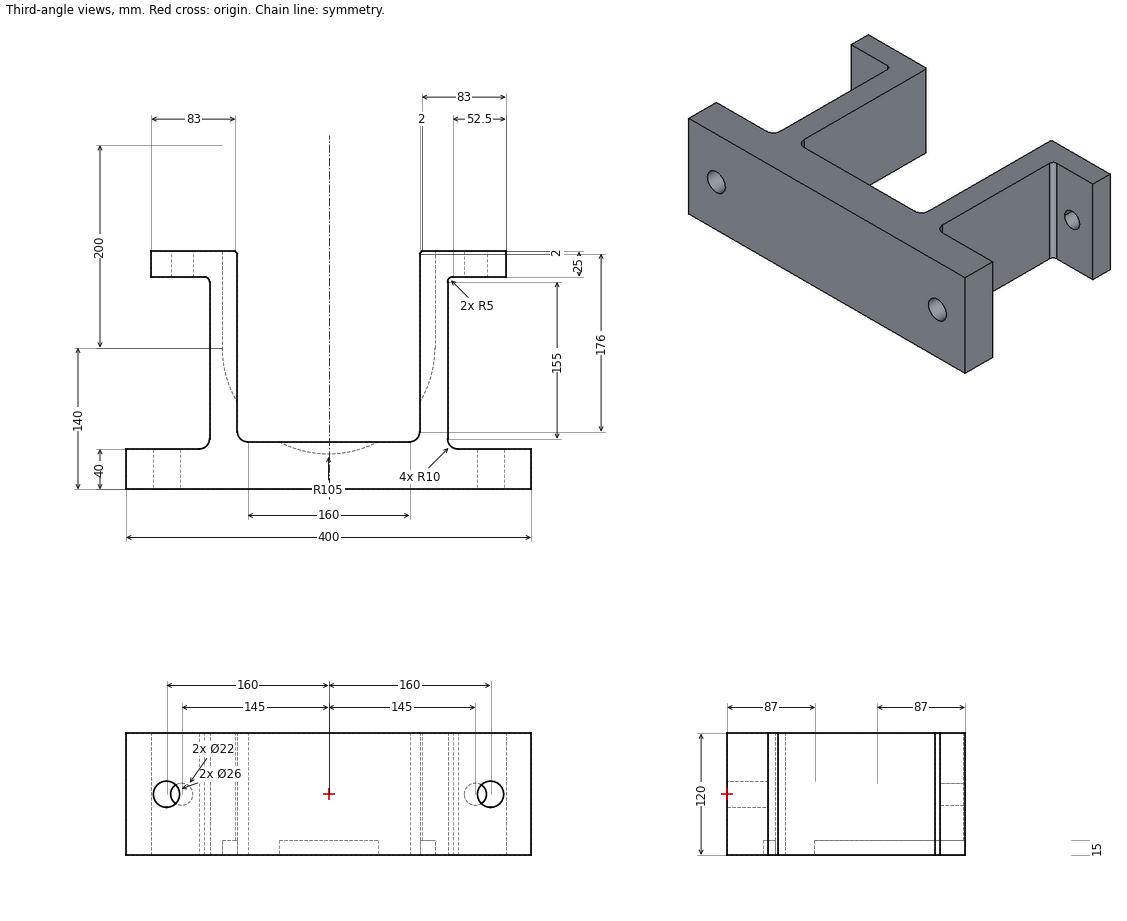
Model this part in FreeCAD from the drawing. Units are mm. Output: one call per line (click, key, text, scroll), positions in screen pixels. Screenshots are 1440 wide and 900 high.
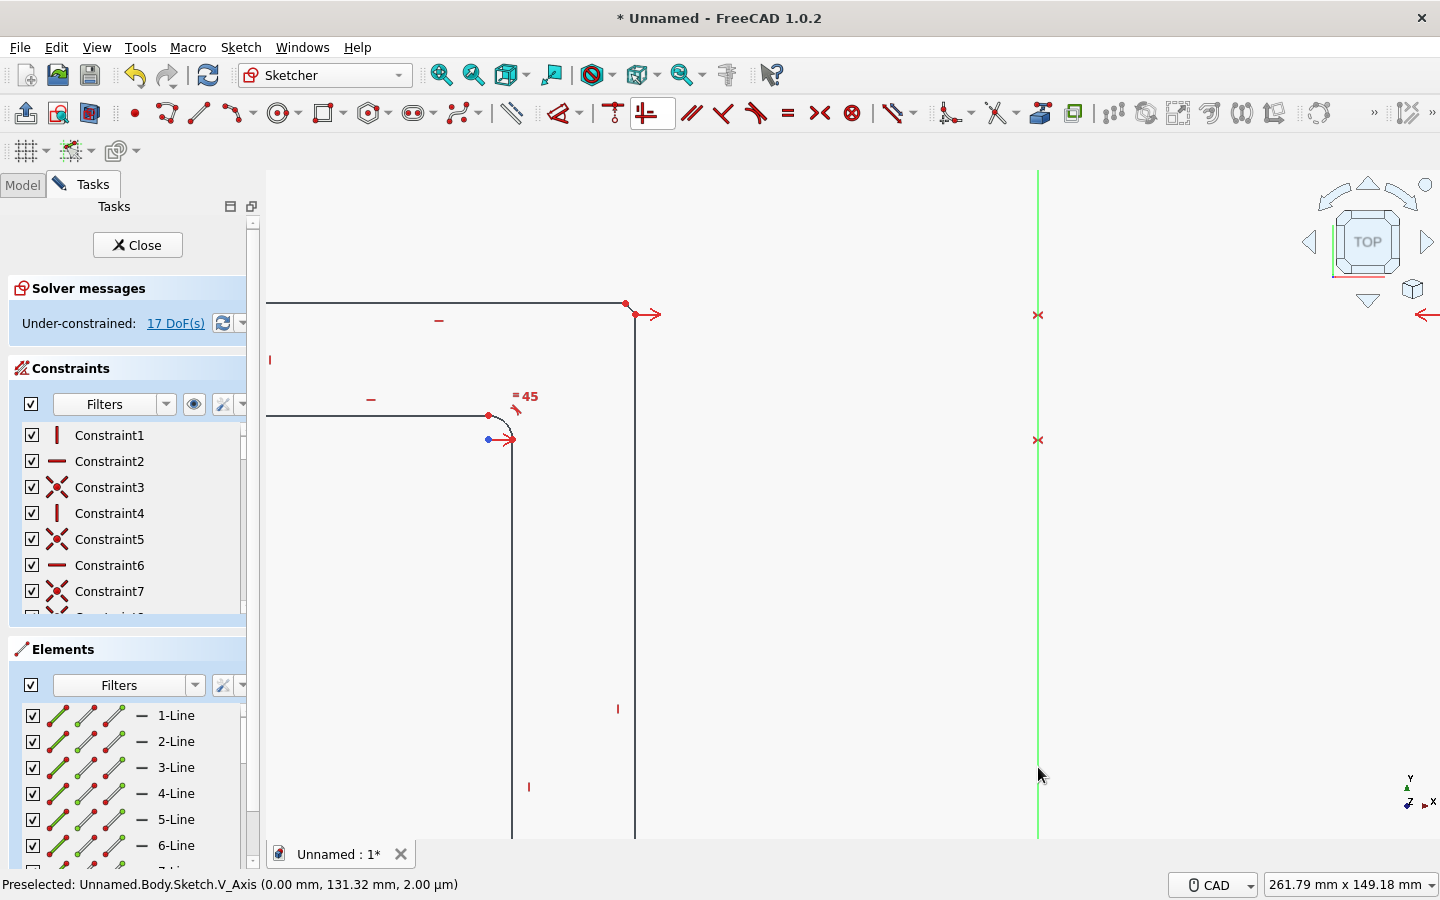
scroll(637, 315, down, 5)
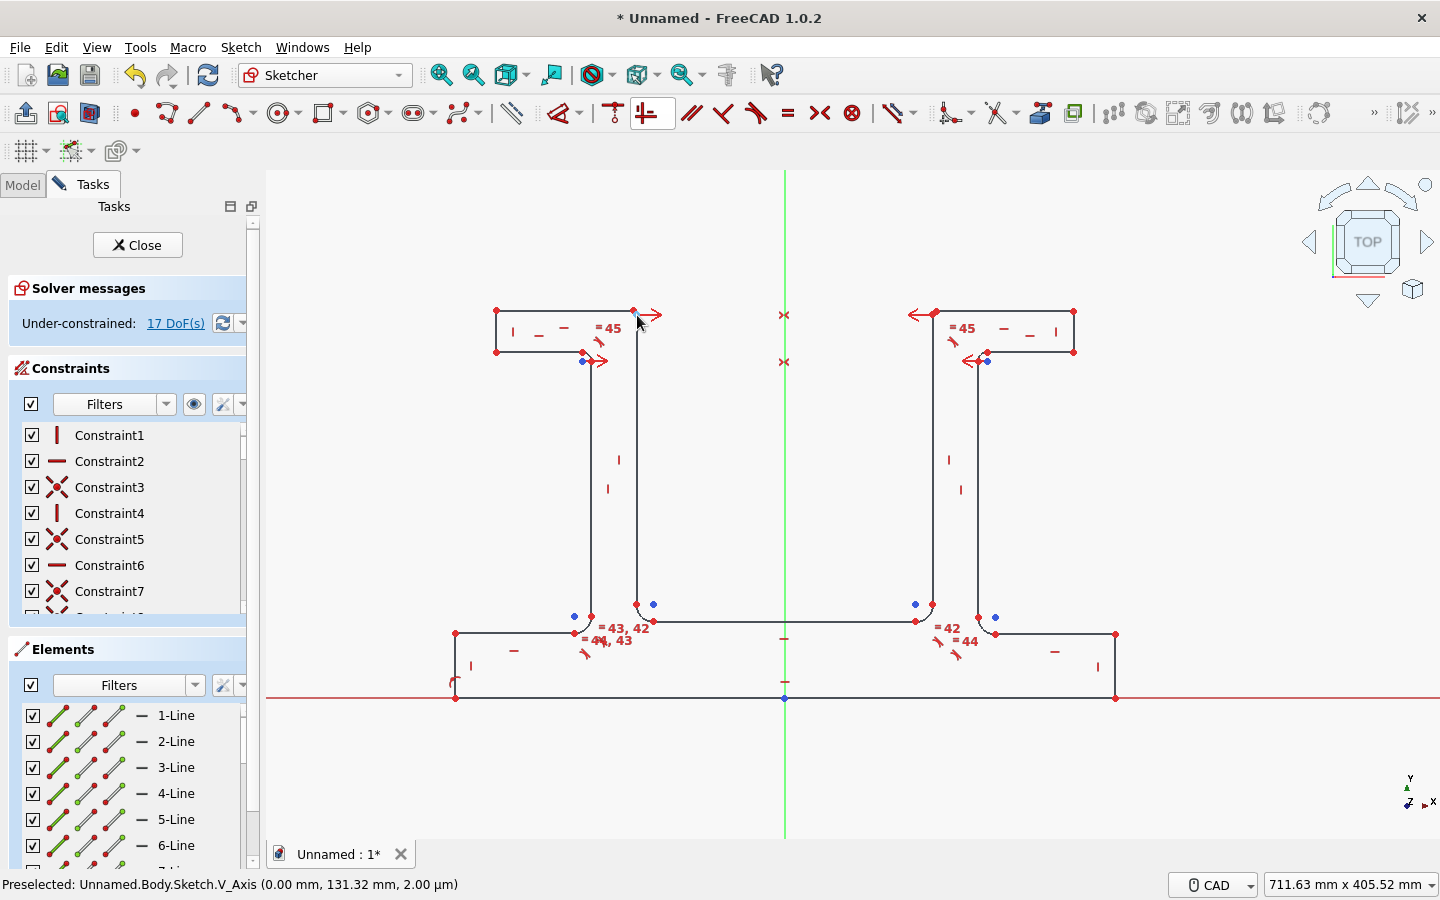
scroll(936, 311, up, 5)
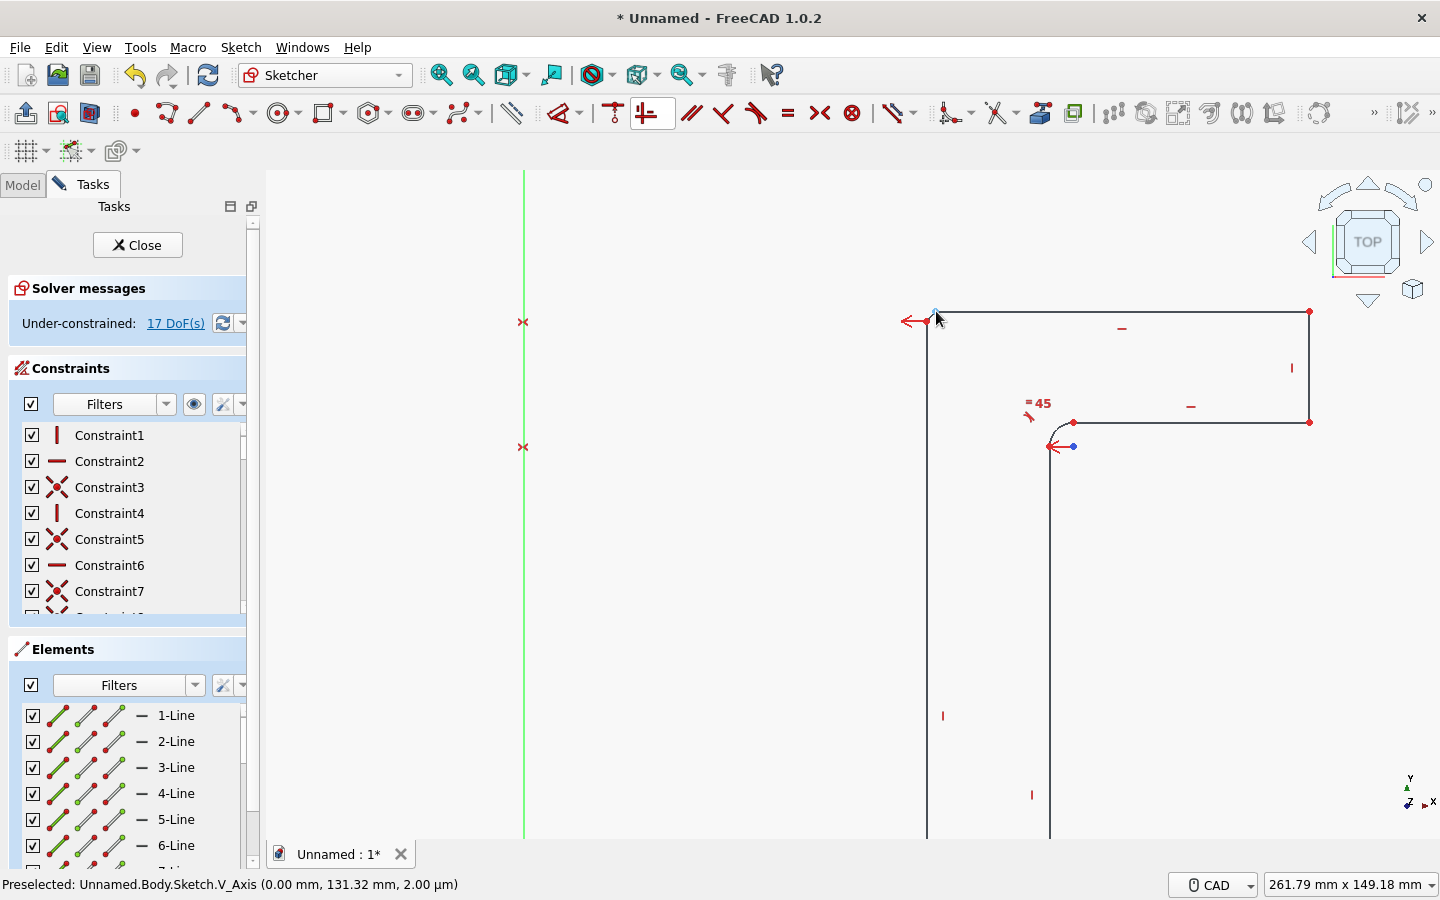
click(936, 312)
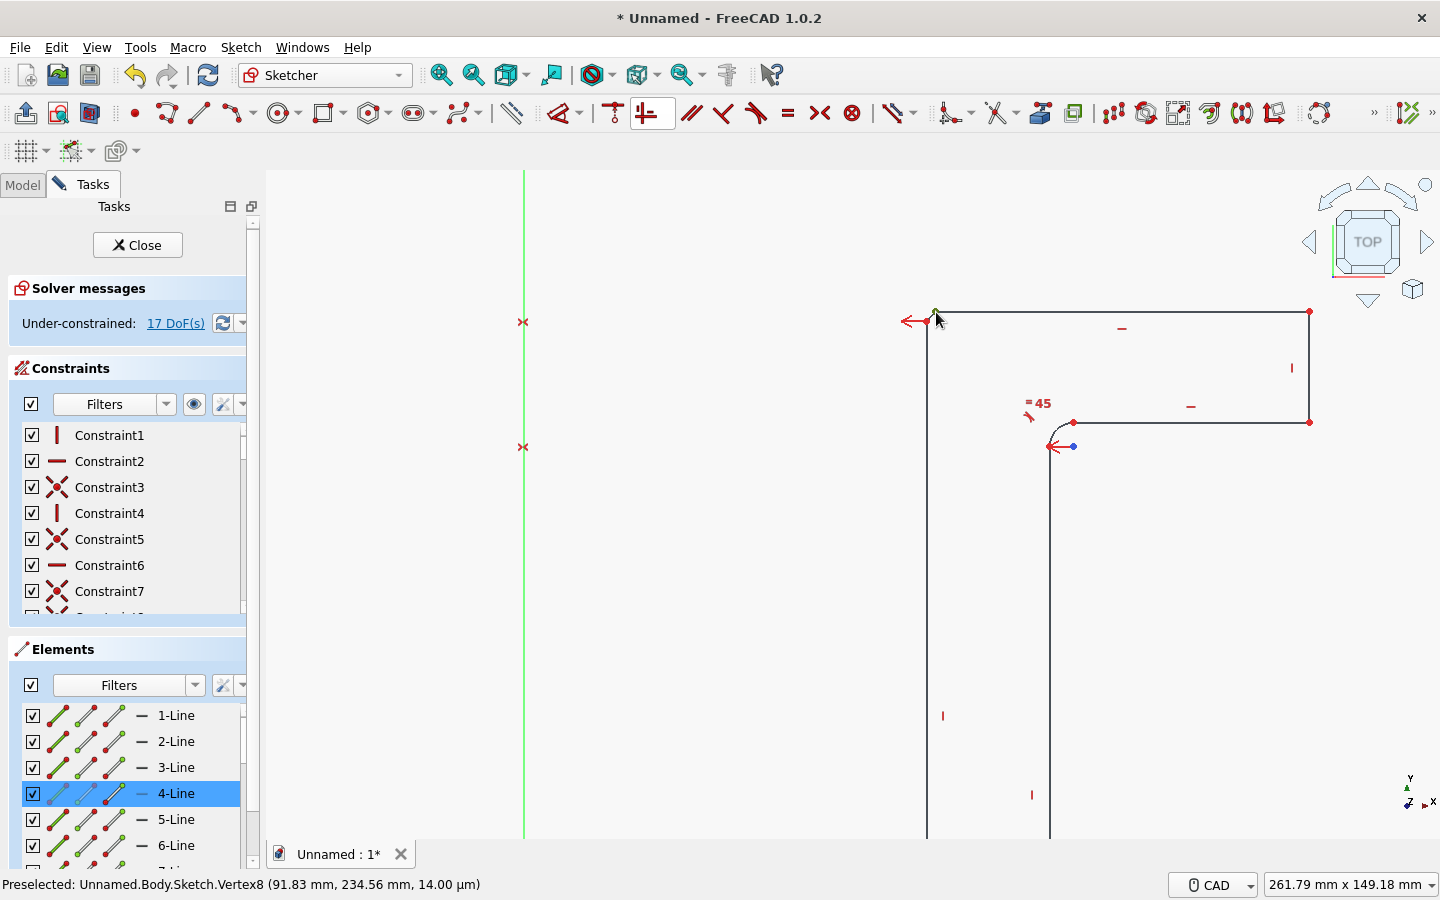
scroll(936, 311, down, 5)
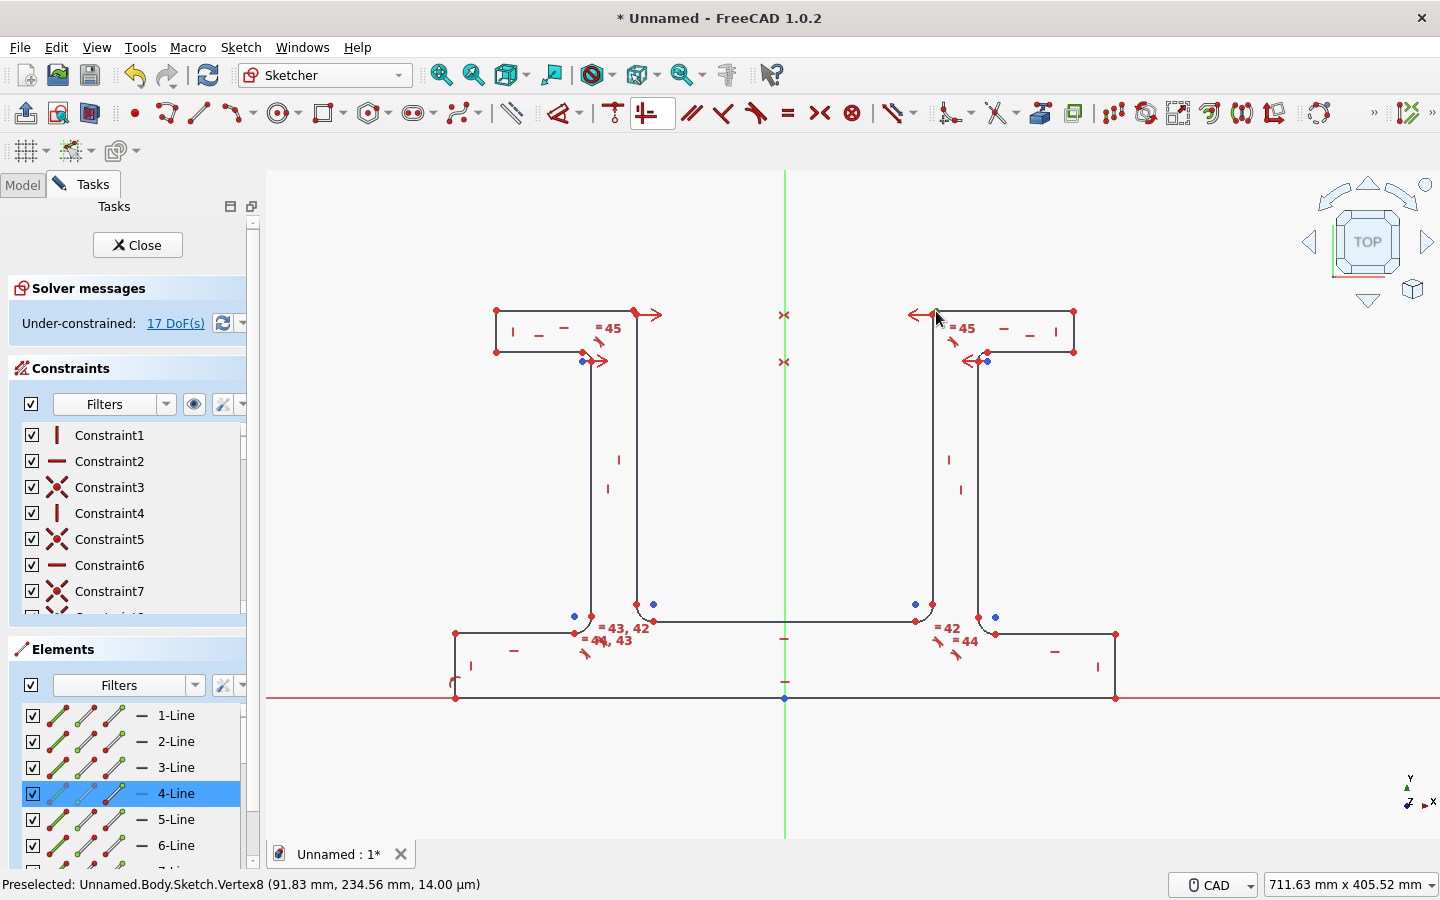
scroll(633, 311, up, 5)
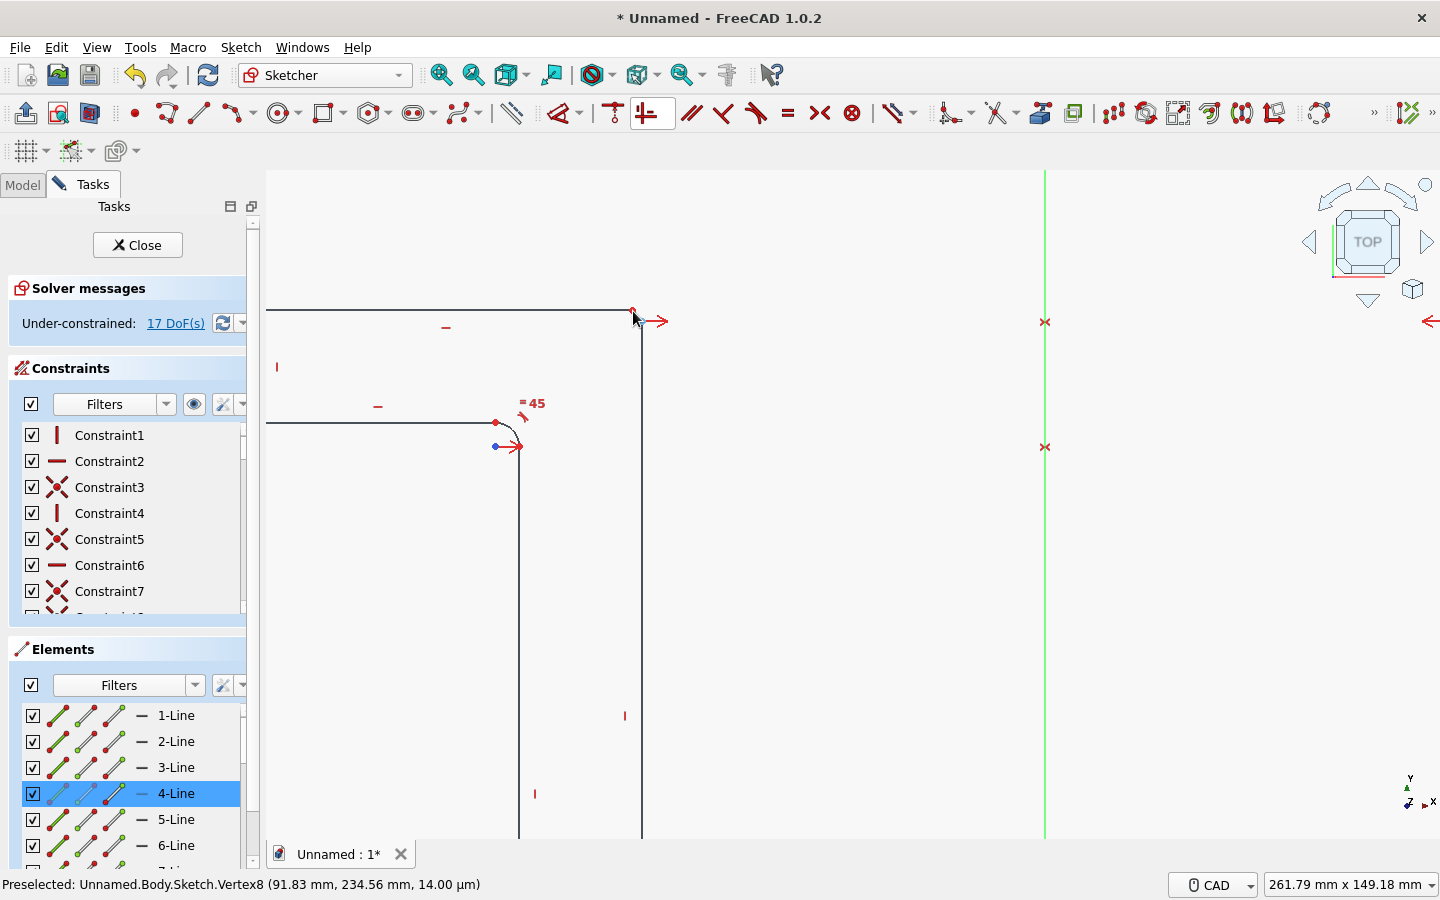
click(633, 310)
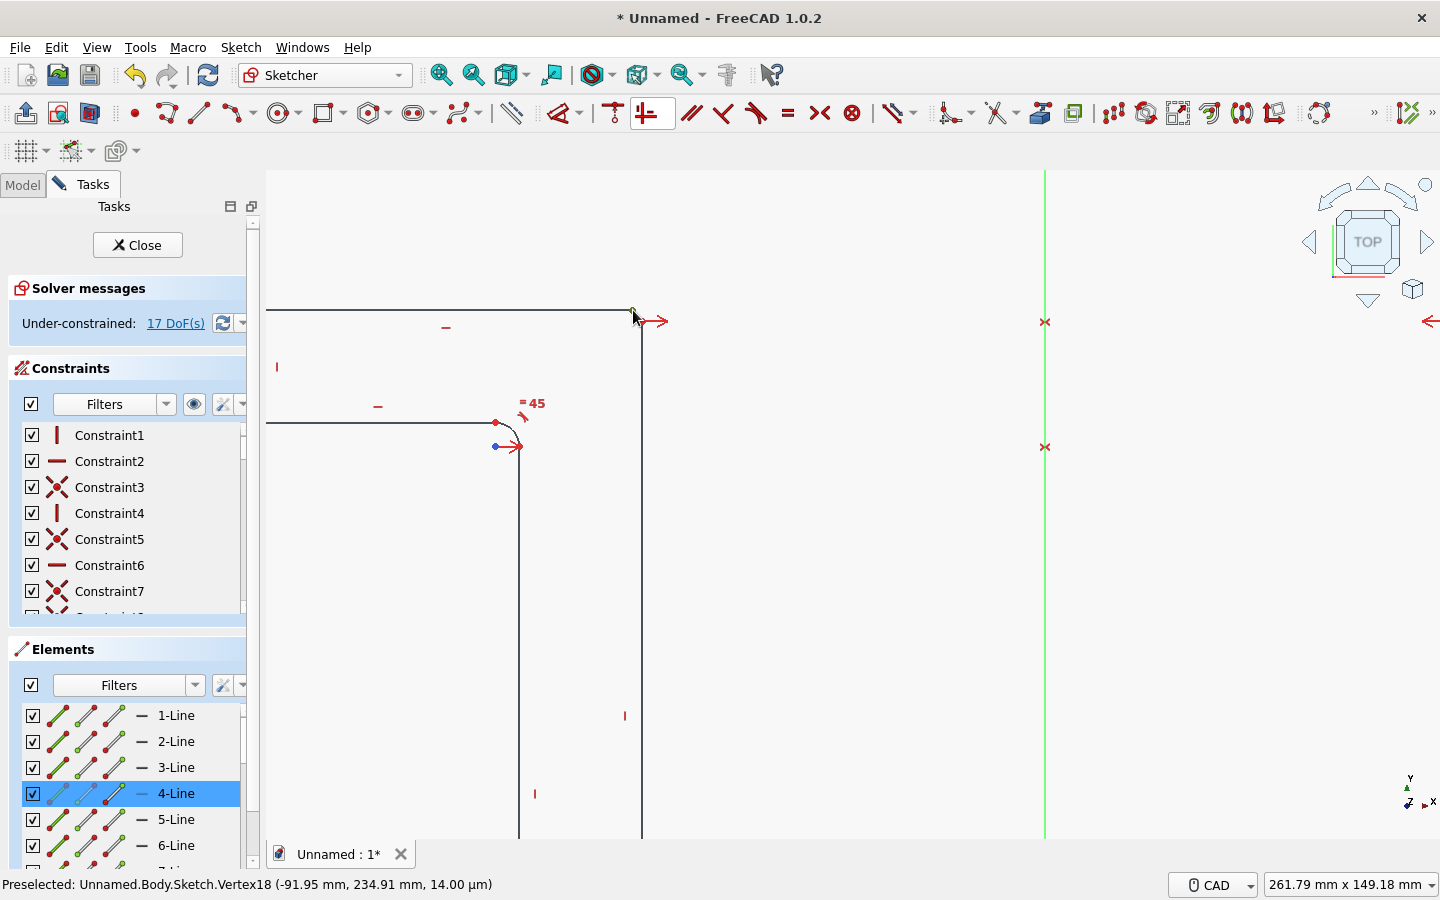
click(1045, 767)